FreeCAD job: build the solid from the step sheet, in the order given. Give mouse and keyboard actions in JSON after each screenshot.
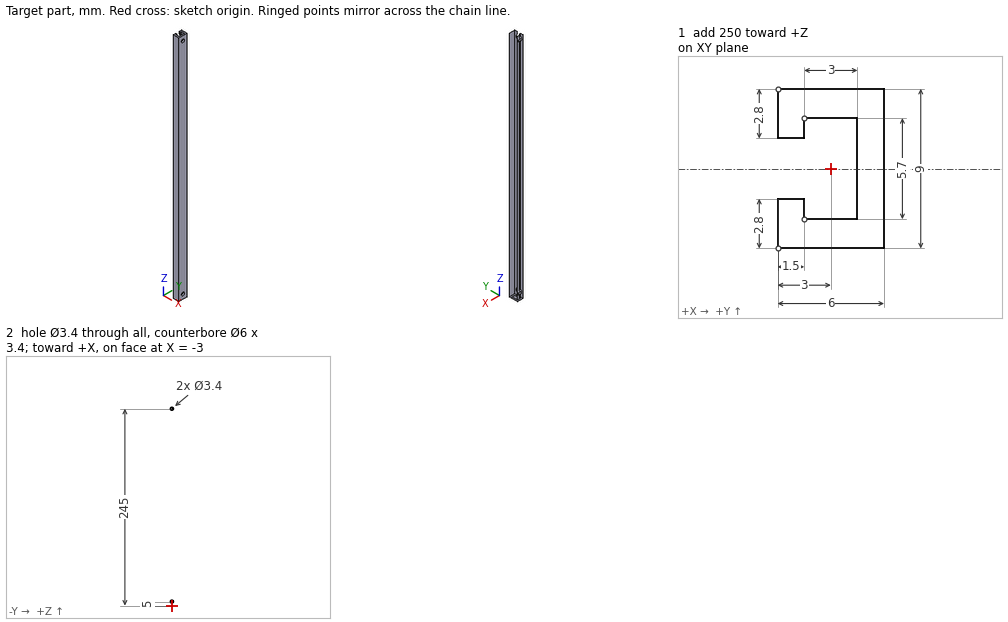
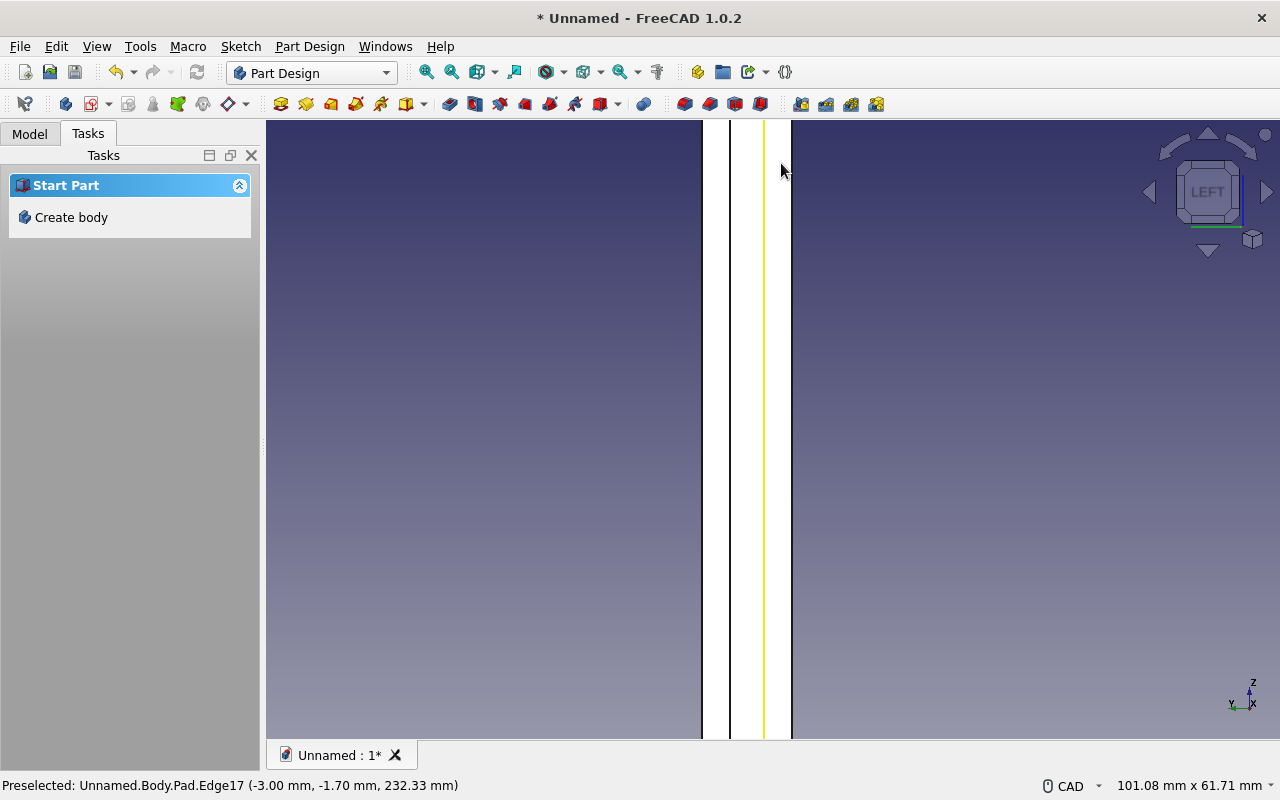
{"action": "left_click", "coordinate": [778, 168]}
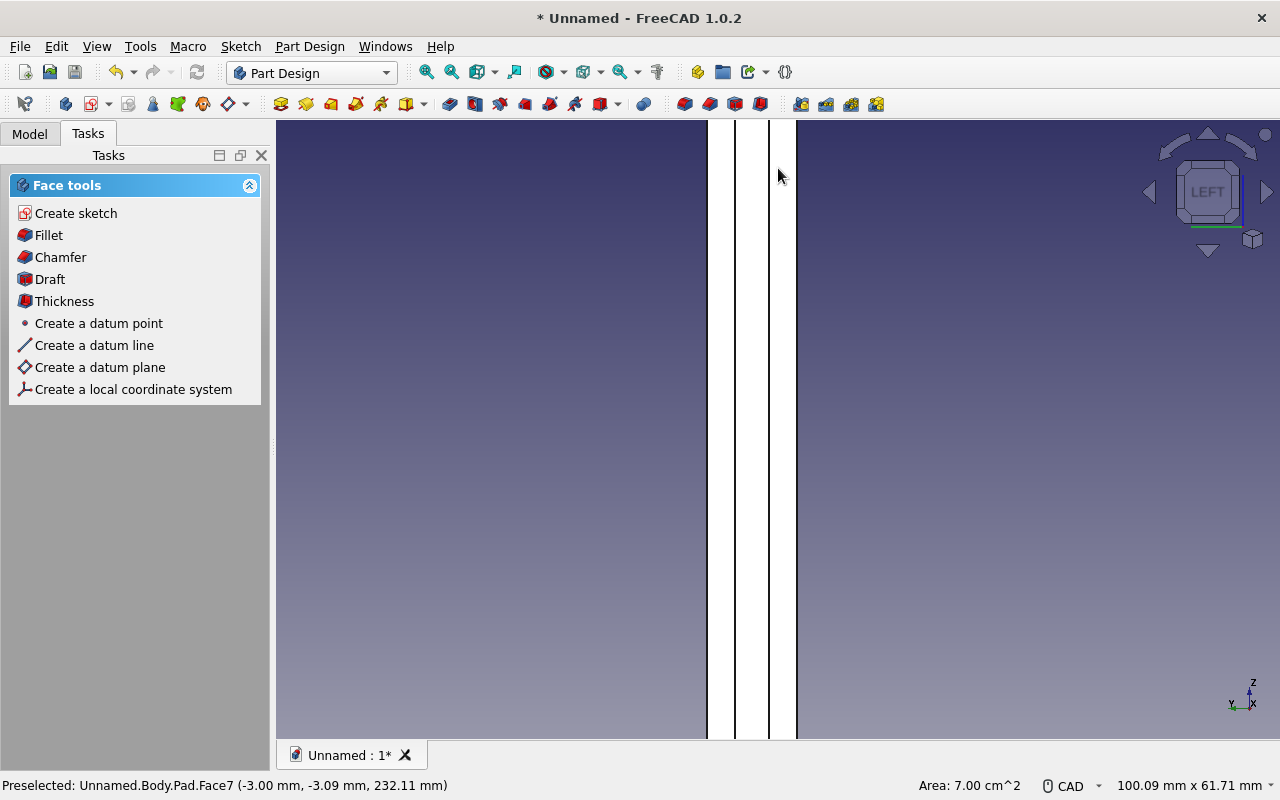
{"action": "left_click", "coordinate": [90, 104]}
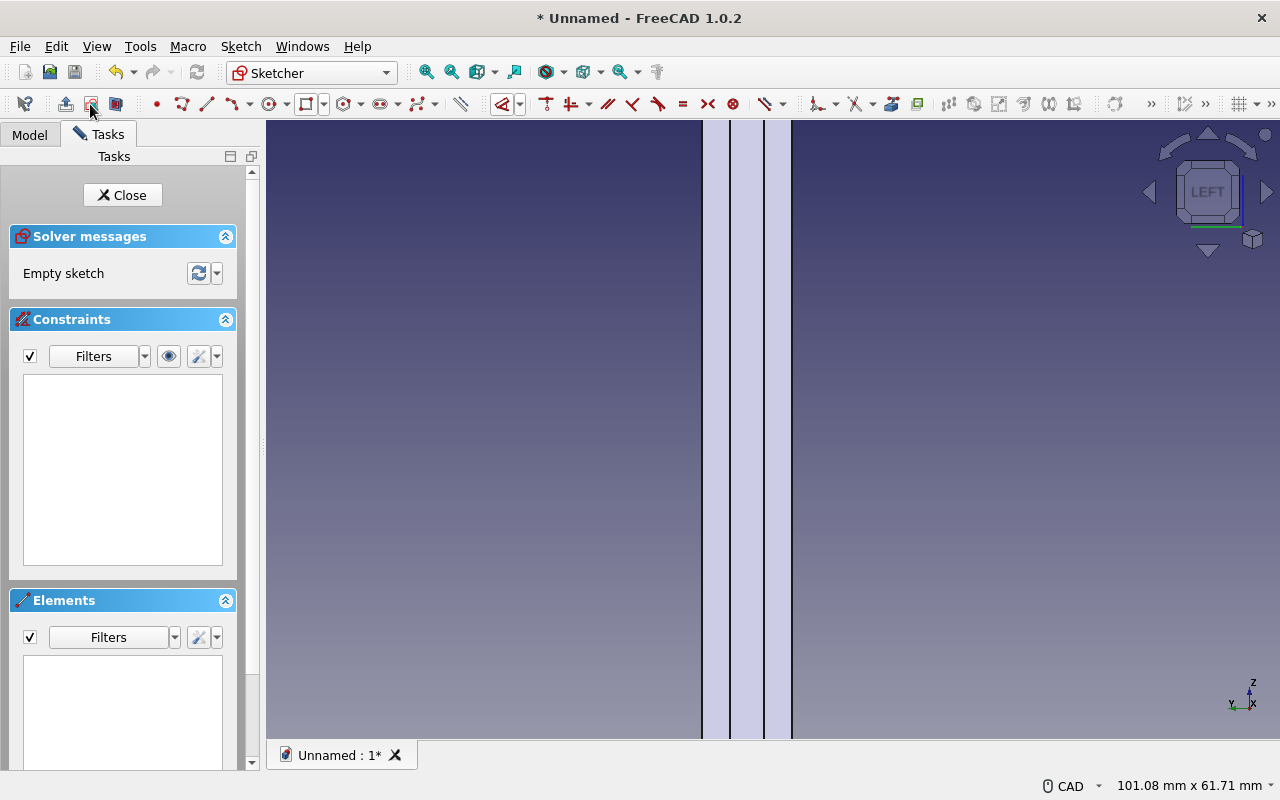
{"action": "scroll", "coordinate": [696, 265], "scroll_direction": "down", "scroll_amount": 9}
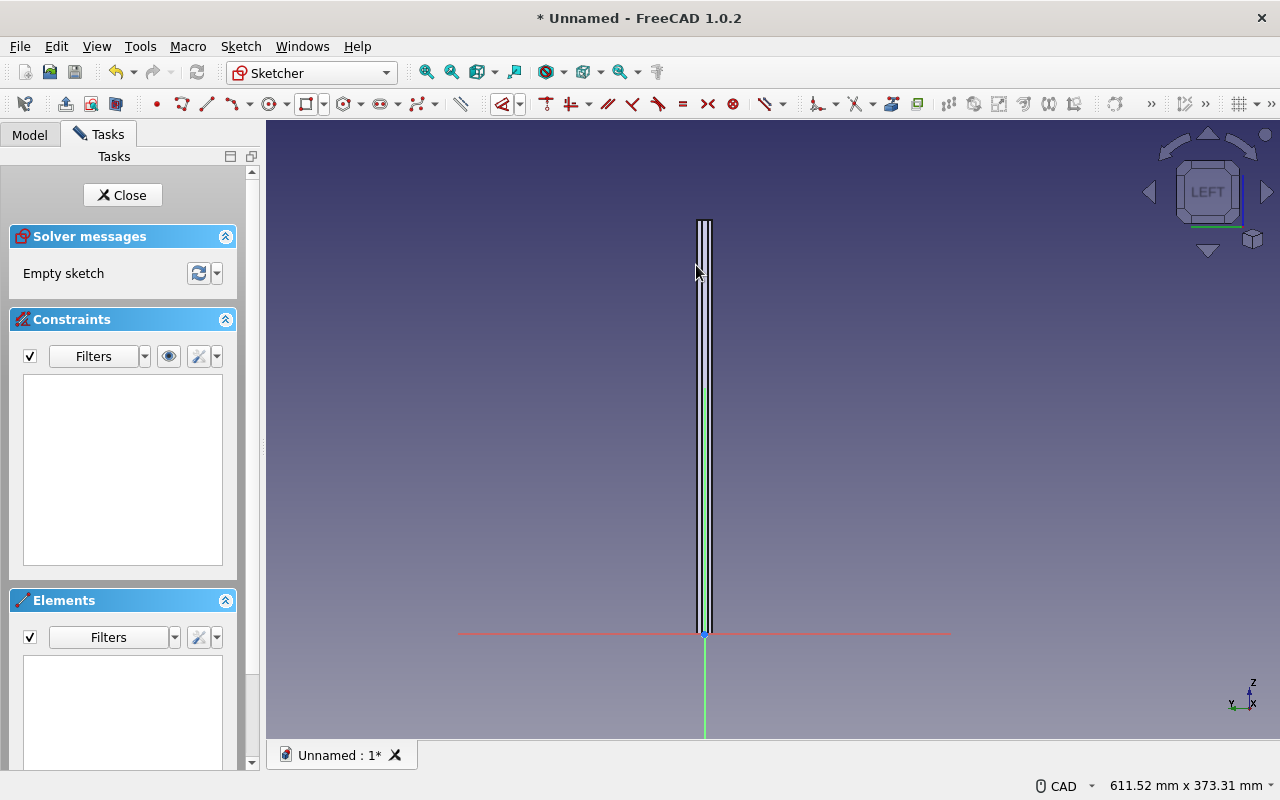
{"action": "key", "text": "g c"}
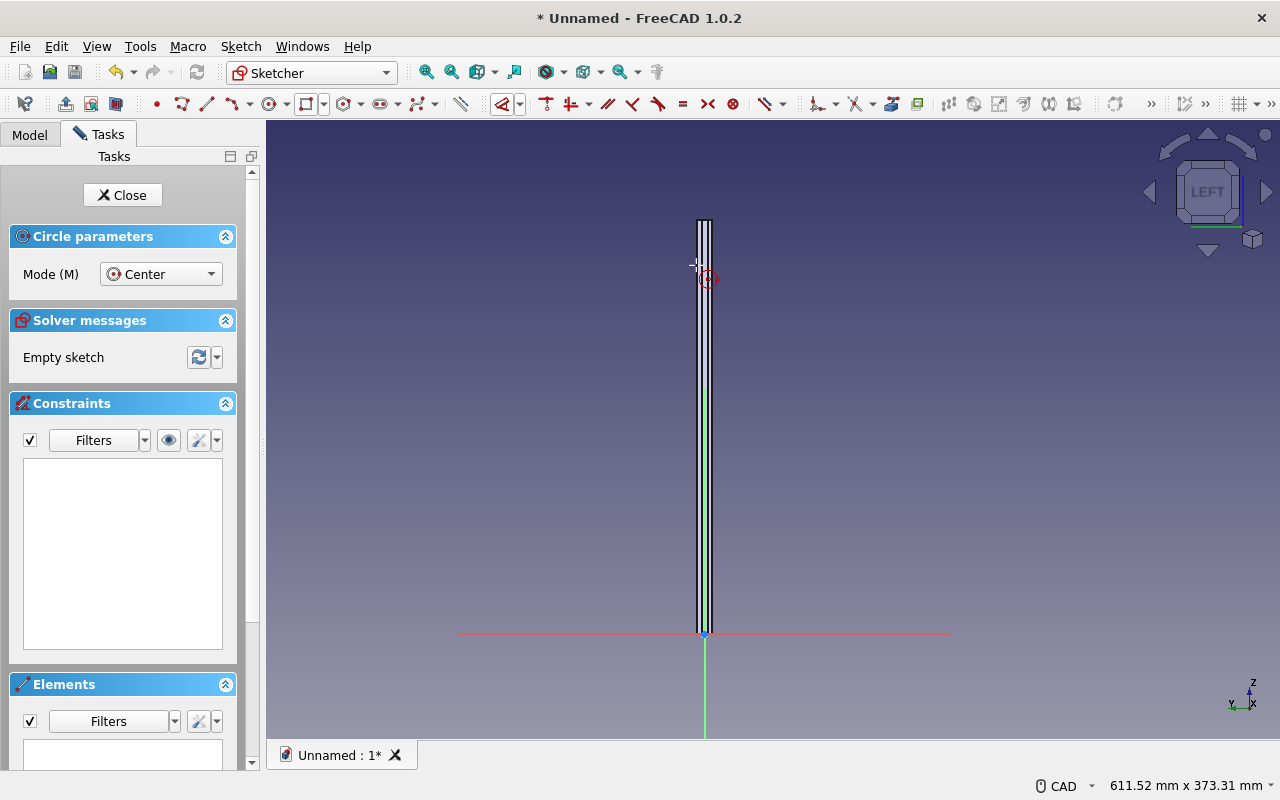
{"action": "scroll", "coordinate": [705, 228], "scroll_direction": "up", "scroll_amount": 11}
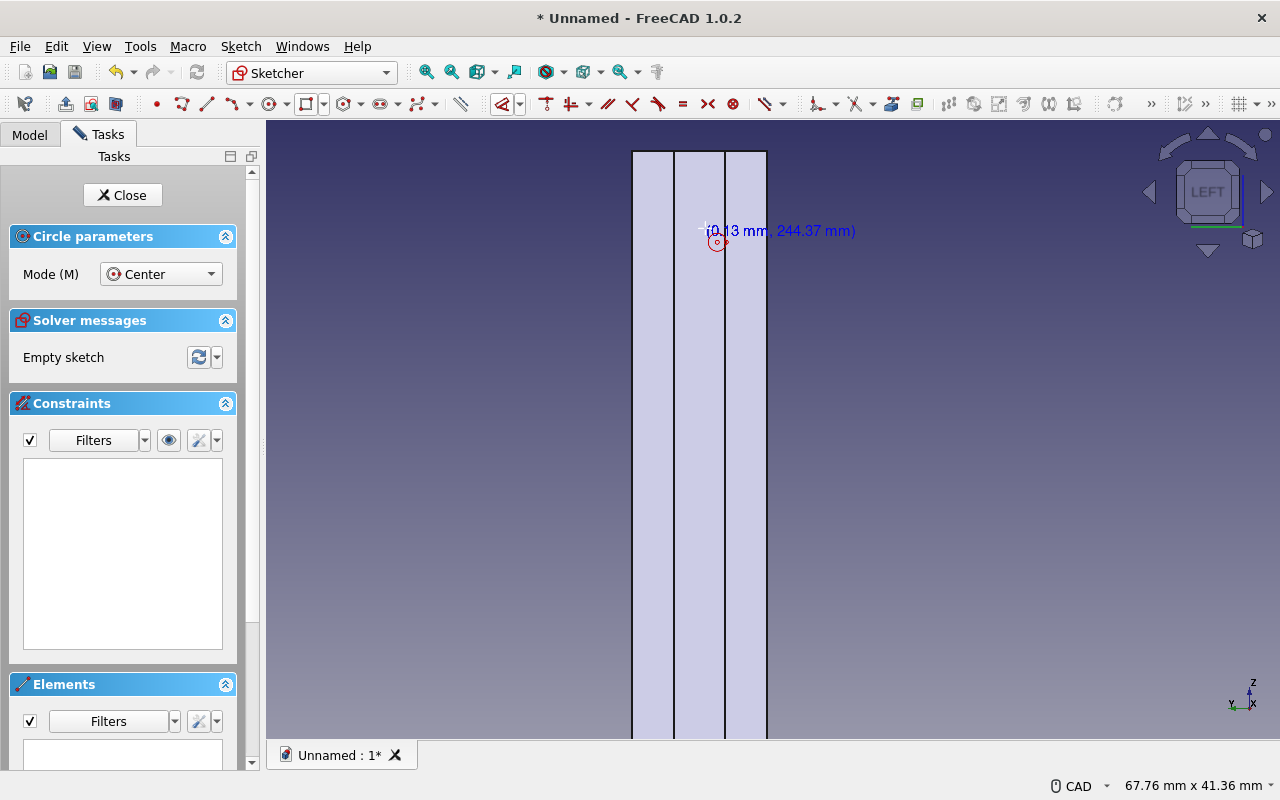
{"action": "scroll", "coordinate": [705, 228], "scroll_direction": "down", "scroll_amount": 11}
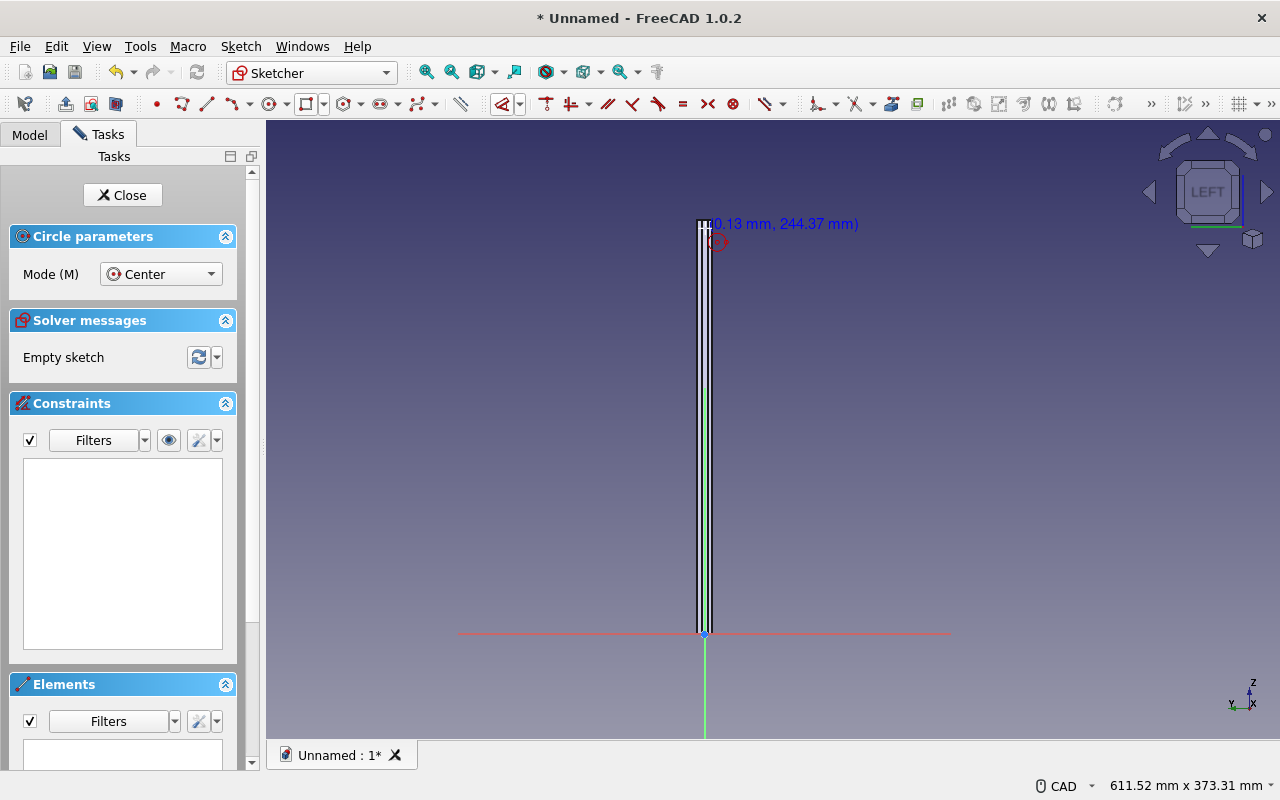
{"action": "left_click", "coordinate": [705, 228]}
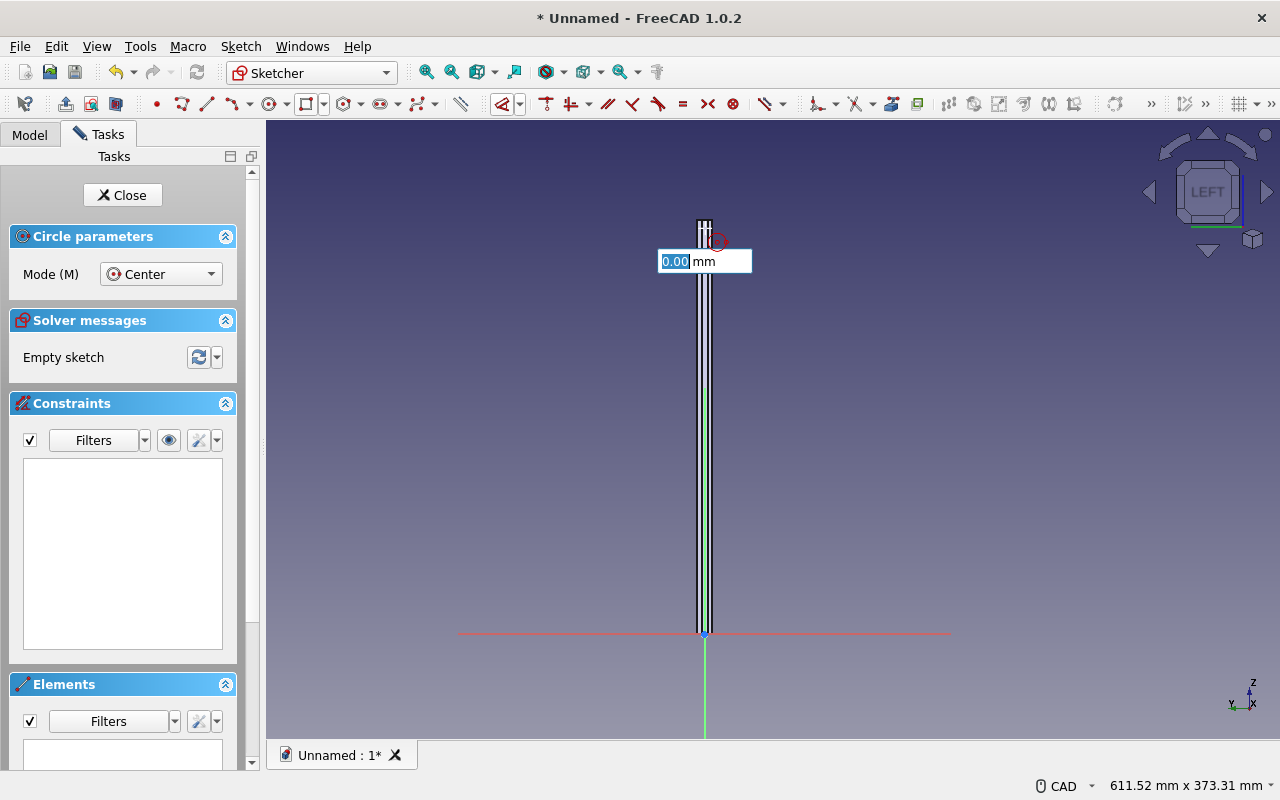
{"action": "scroll", "coordinate": [707, 227], "scroll_direction": "up", "scroll_amount": 9}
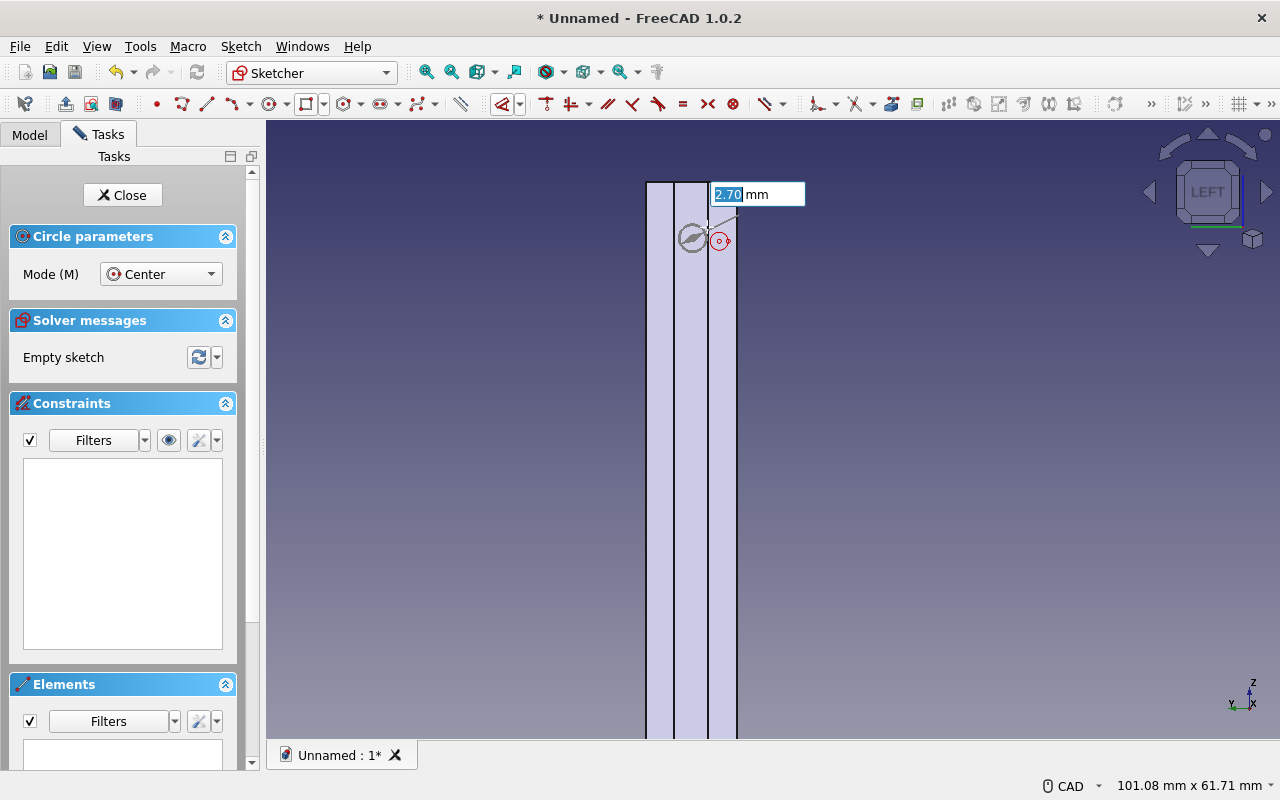
{"action": "left_click", "coordinate": [707, 226]}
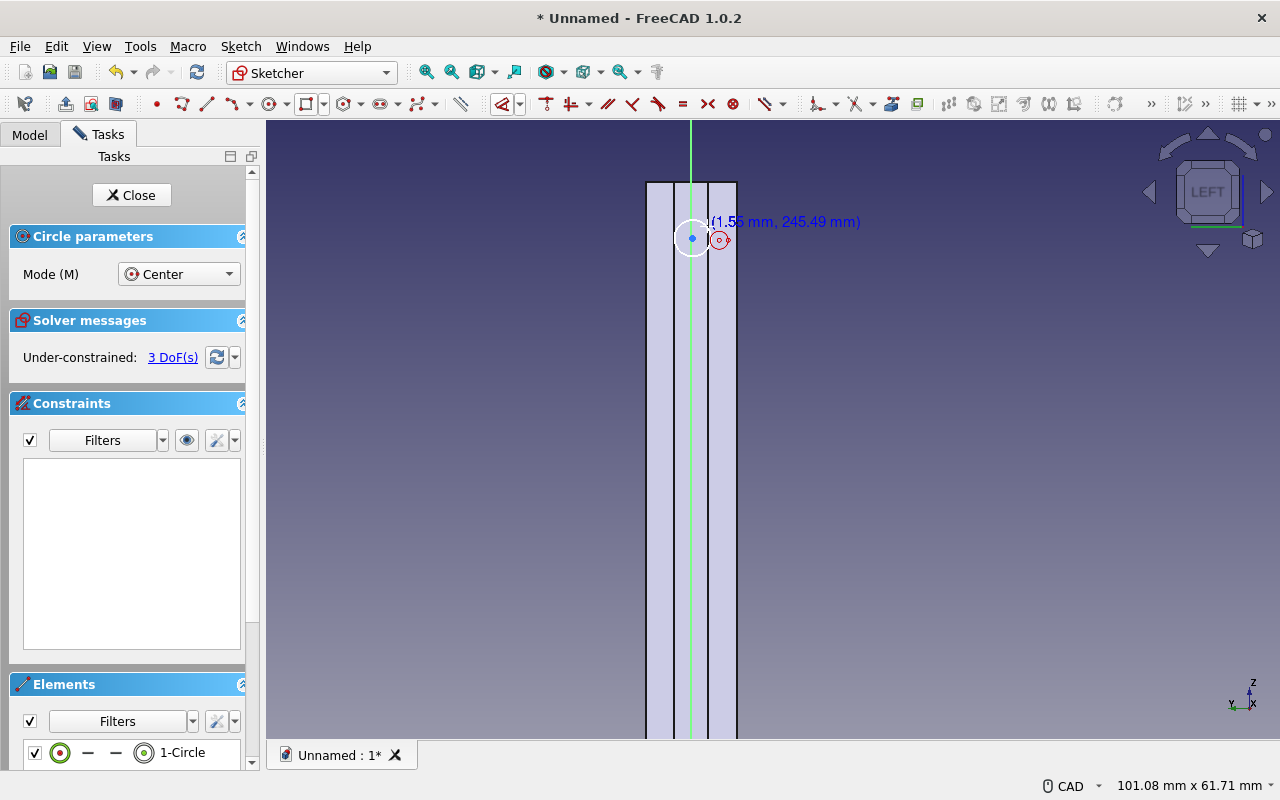
{"action": "scroll", "coordinate": [707, 227], "scroll_direction": "down", "scroll_amount": 9}